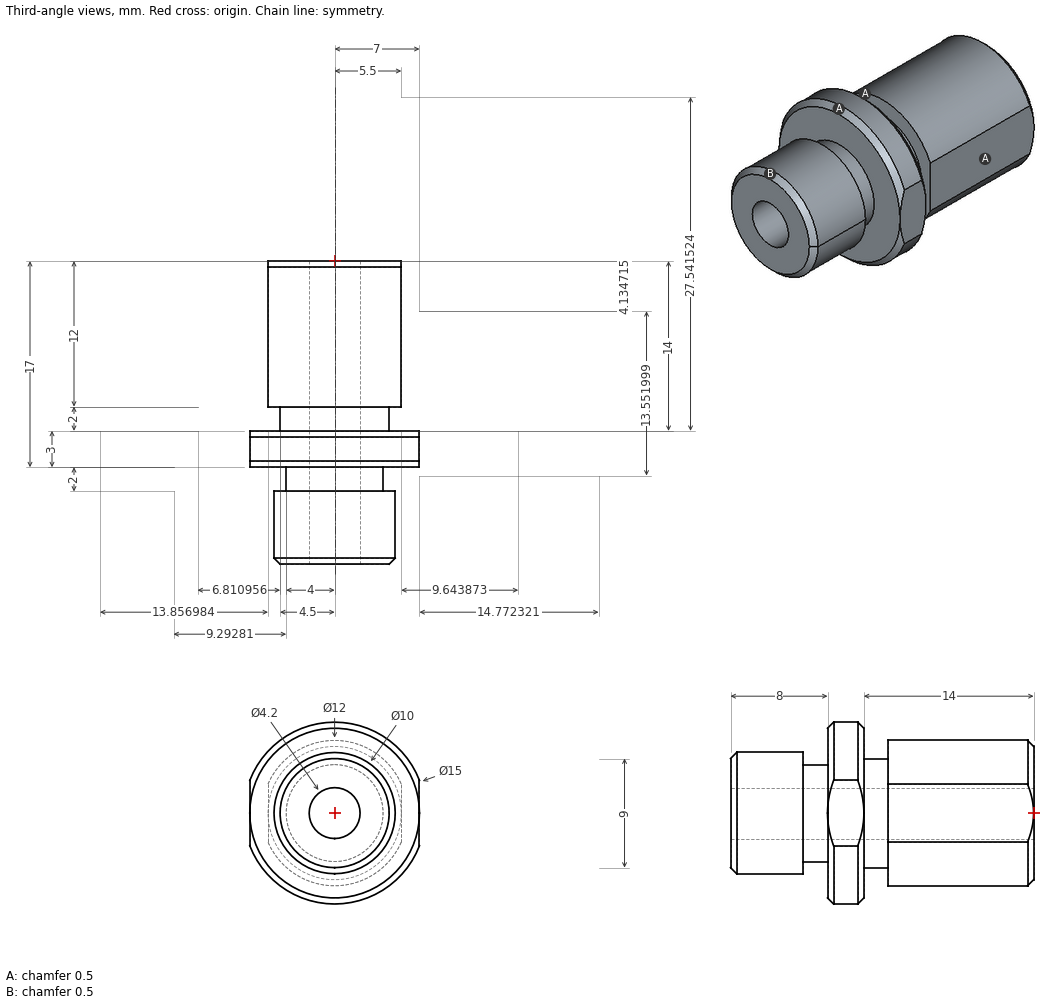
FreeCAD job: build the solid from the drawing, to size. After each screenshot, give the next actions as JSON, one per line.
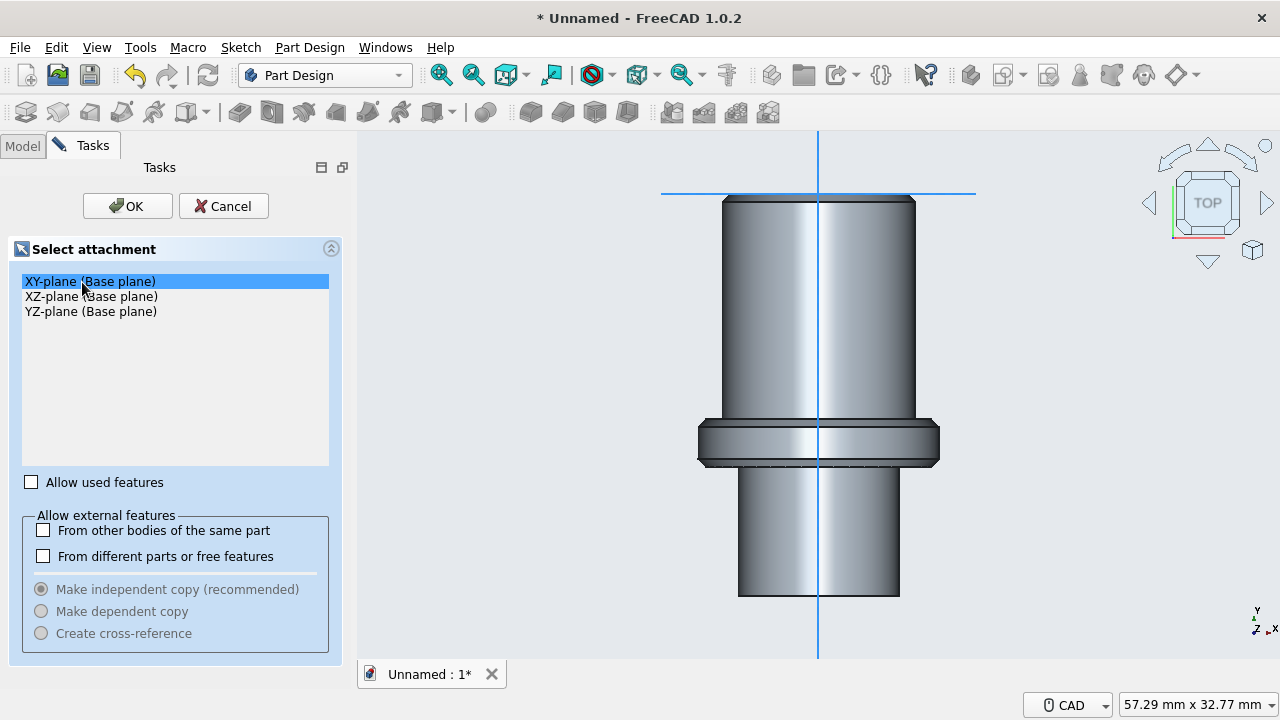
{"action": "left_click", "coordinate": [128, 206]}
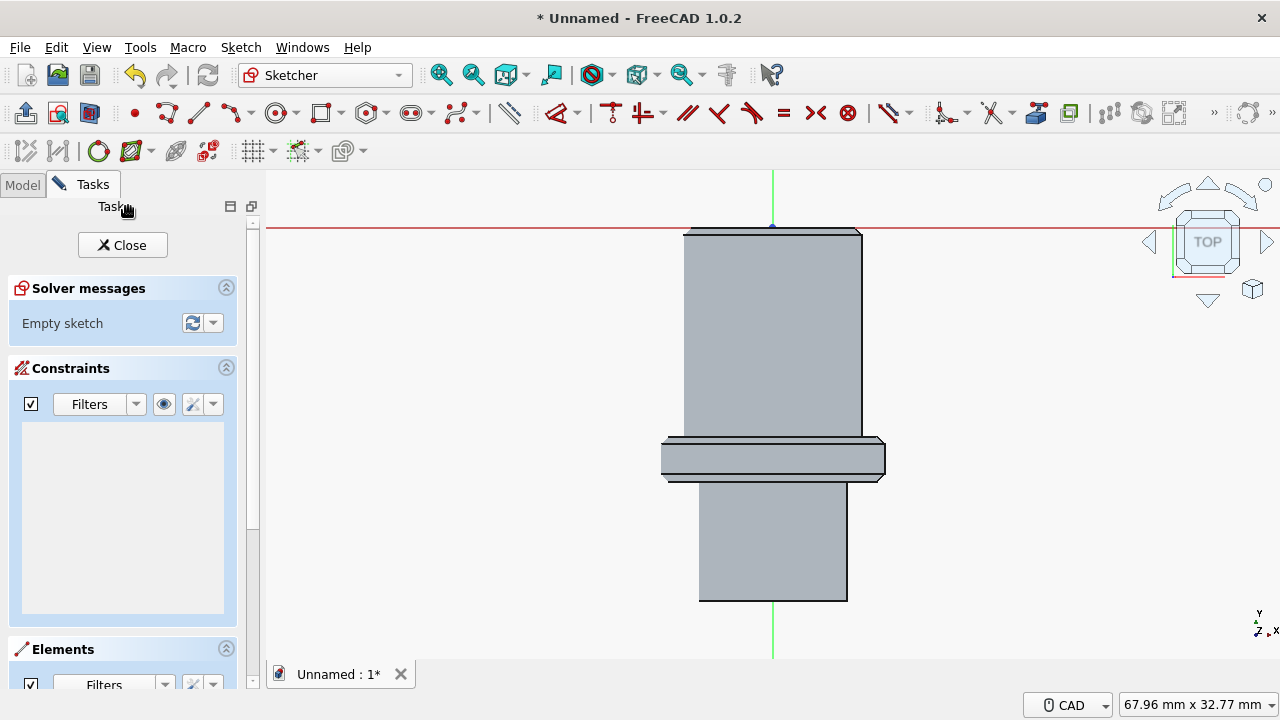
{"action": "key", "text": "q s"}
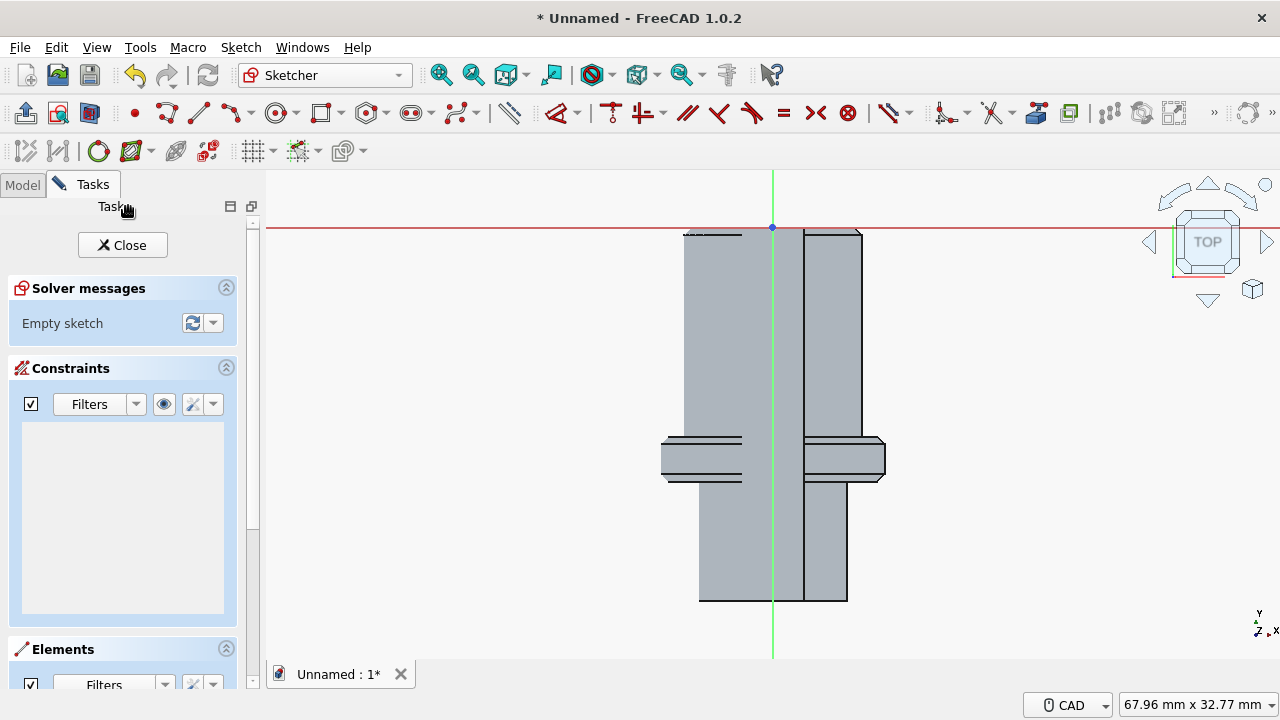
{"action": "scroll", "coordinate": [294, 631], "scroll_direction": "down", "scroll_amount": 1}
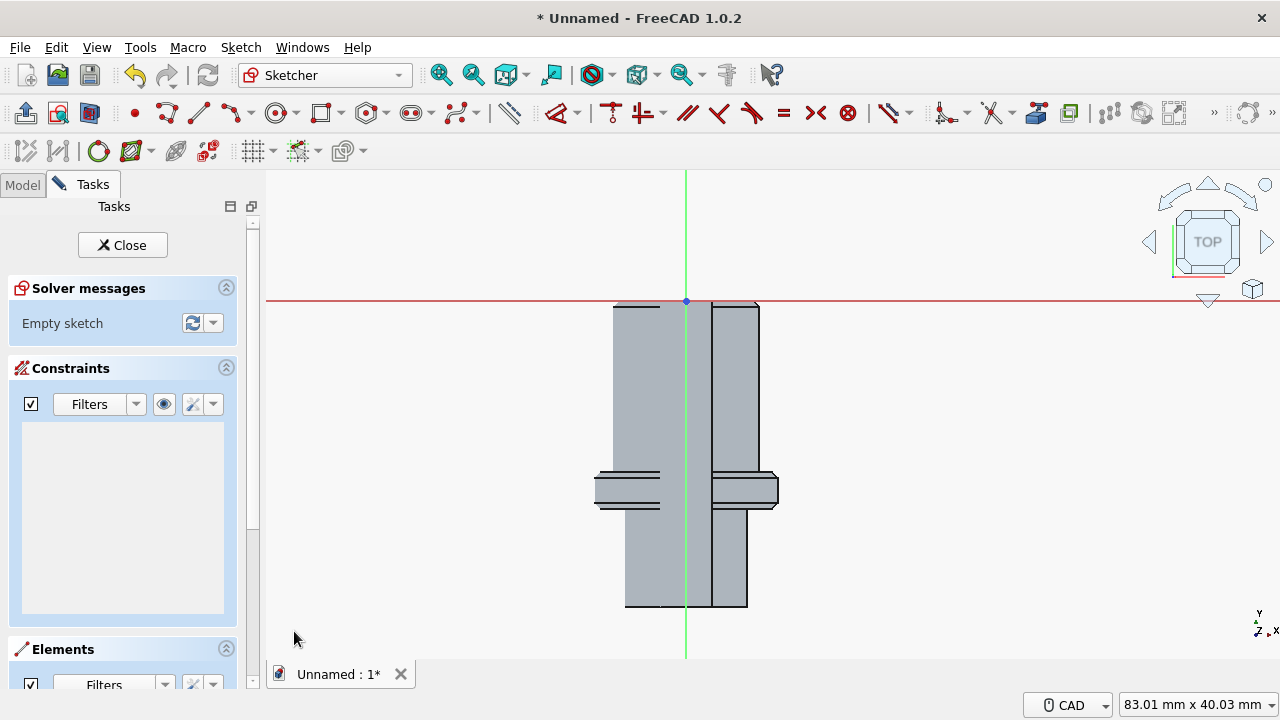
{"action": "scroll", "coordinate": [1052, 399], "scroll_direction": "up", "scroll_amount": 2}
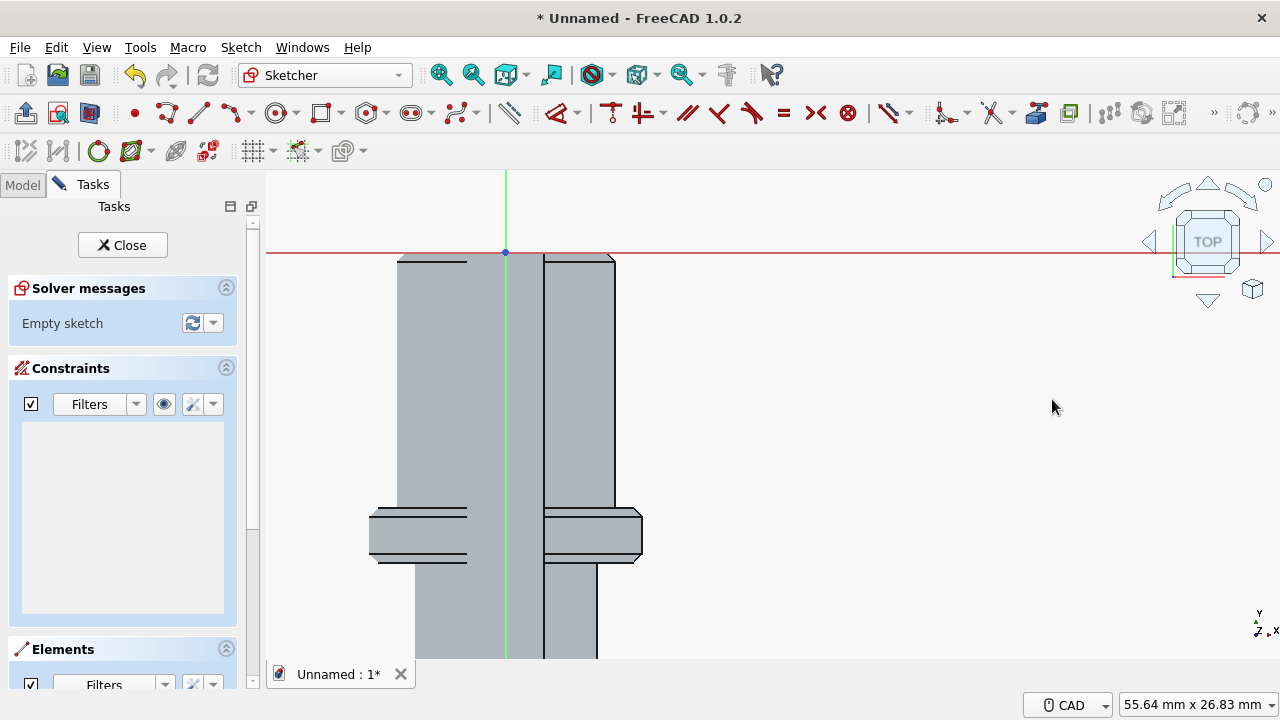
{"action": "left_click", "coordinate": [322, 114]}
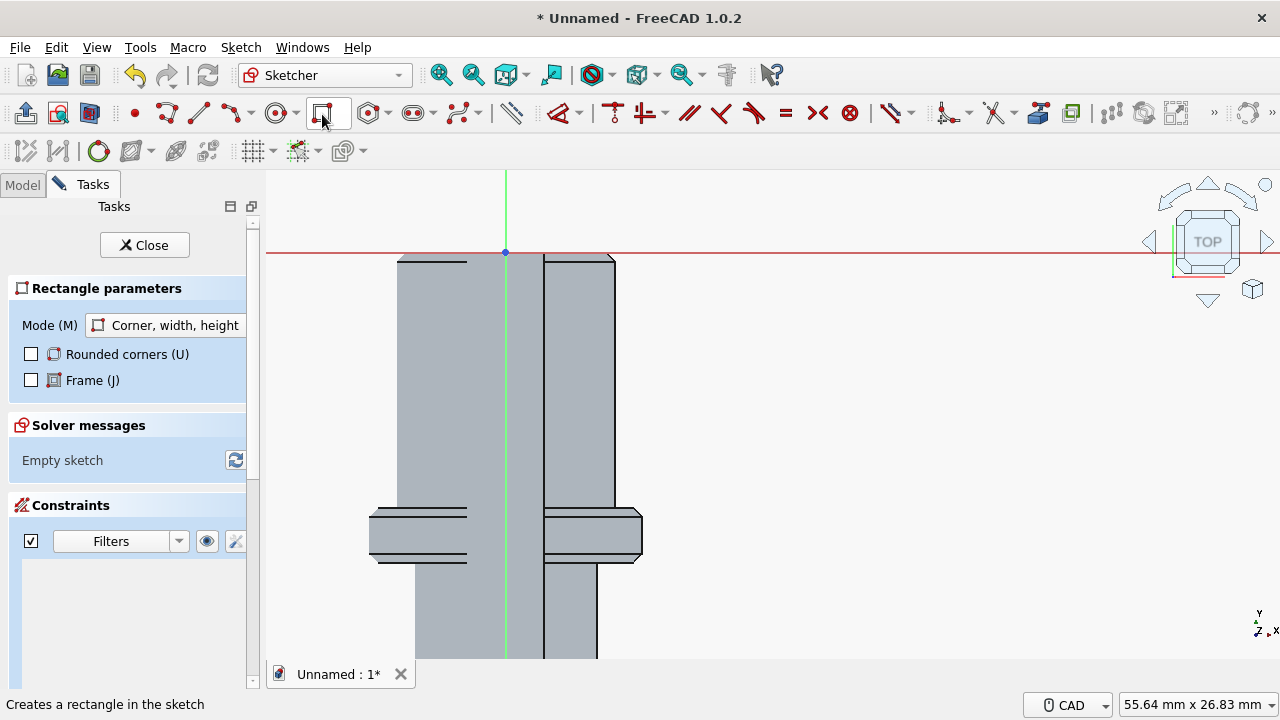
{"action": "left_click", "coordinate": [633, 328]}
{"action": "left_click", "coordinate": [902, 575]}
{"action": "key", "text": "Escape"}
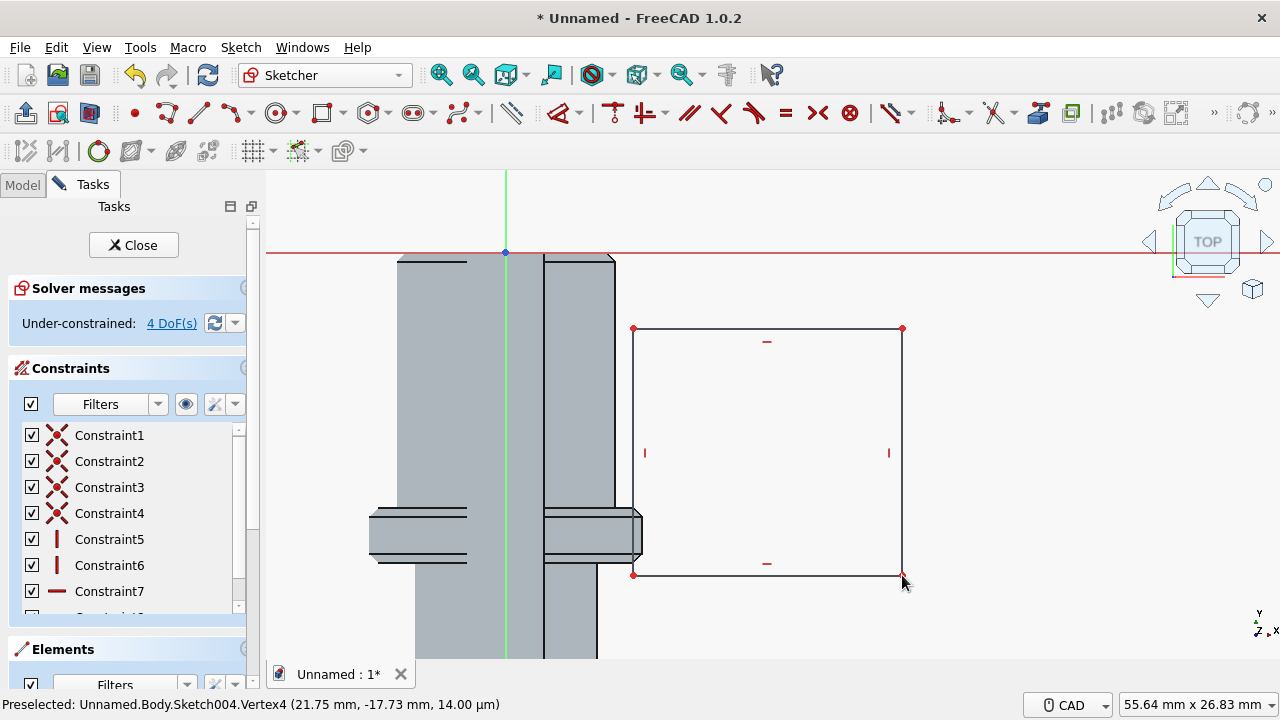
{"action": "key", "text": "d"}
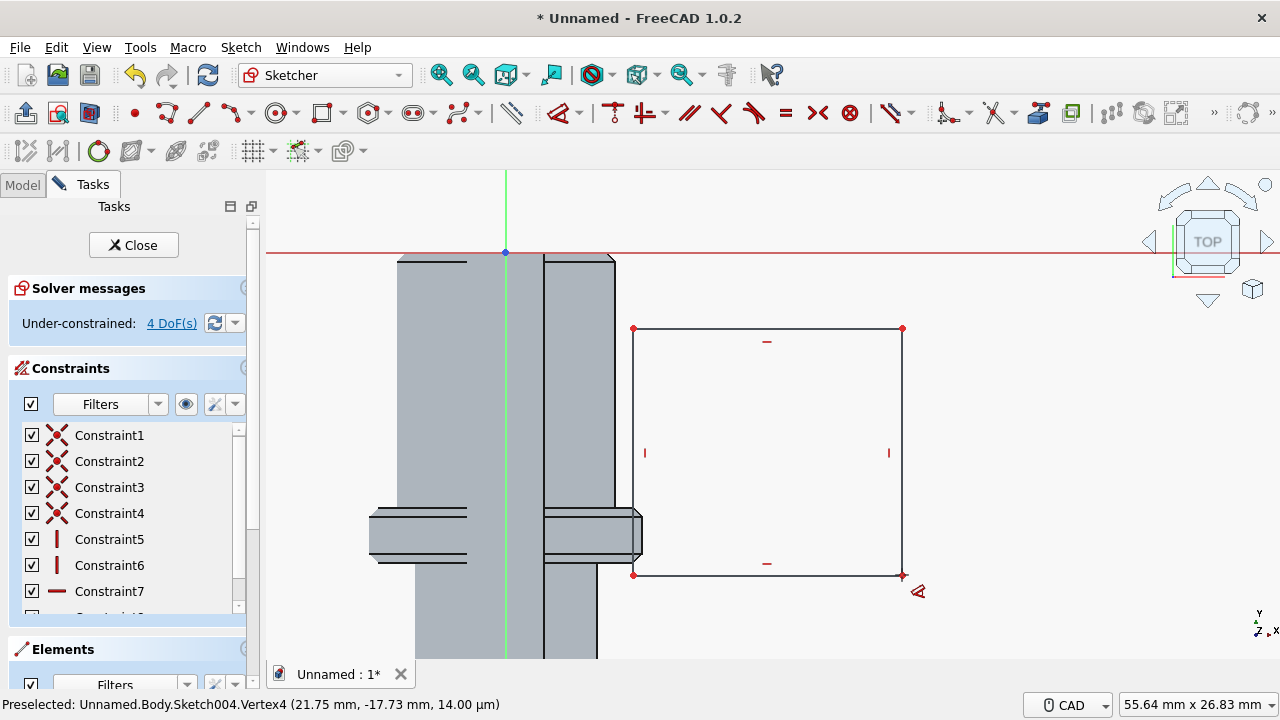
{"action": "left_click", "coordinate": [633, 329]}
{"action": "left_click", "coordinate": [569, 219]}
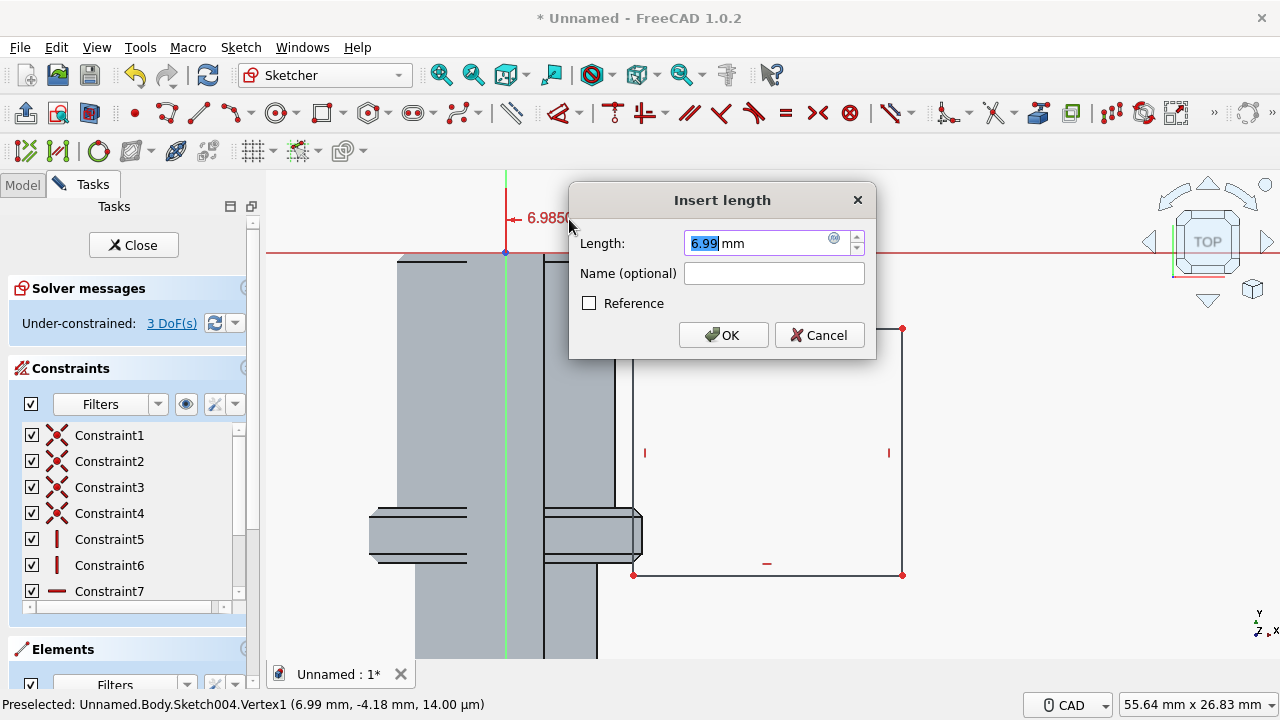
{"action": "type", "text": "7"}
{"action": "key", "text": "Return"}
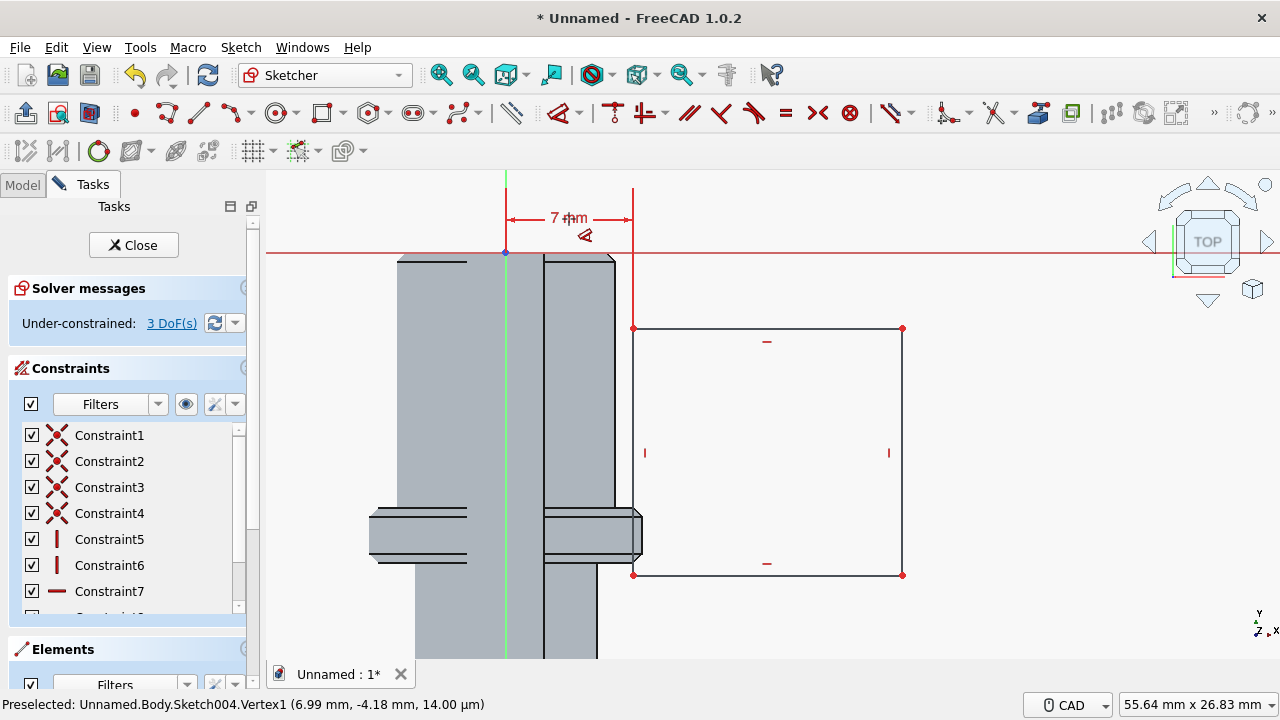
{"action": "left_click", "coordinate": [633, 403]}
{"action": "left_click", "coordinate": [599, 453]}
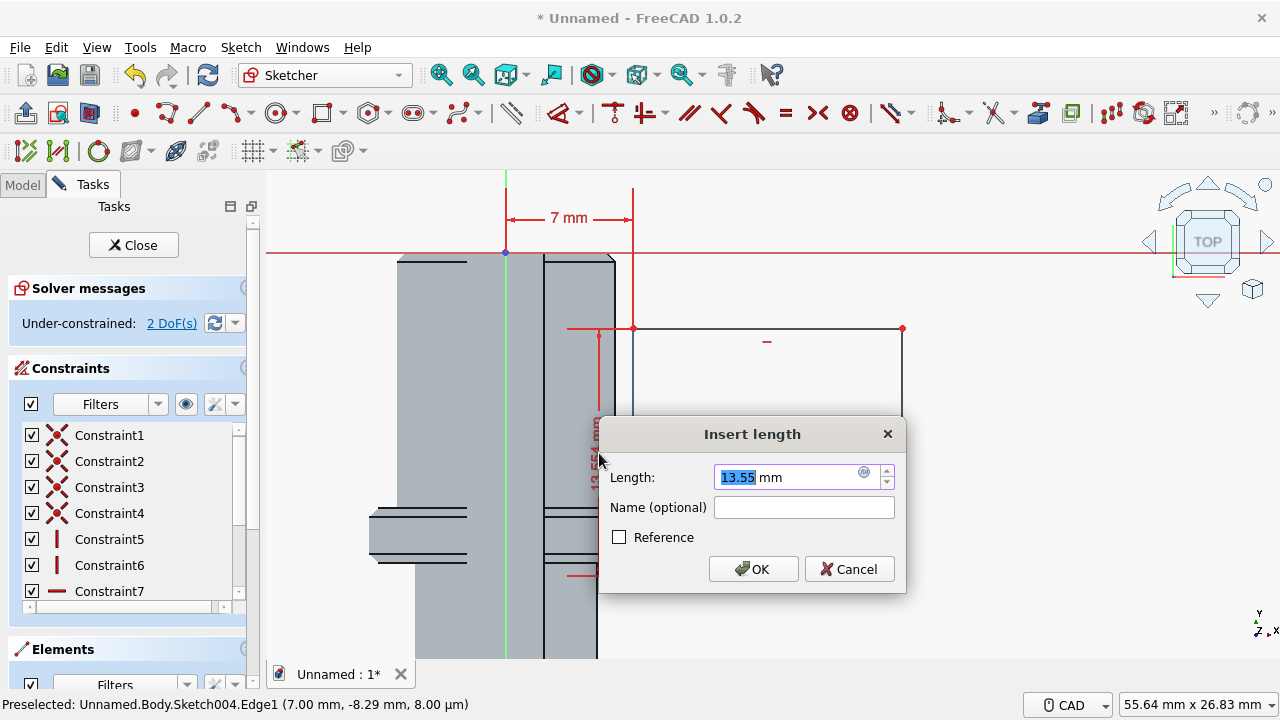
{"action": "type", "text": "13.551999"}
{"action": "key", "text": "Return"}